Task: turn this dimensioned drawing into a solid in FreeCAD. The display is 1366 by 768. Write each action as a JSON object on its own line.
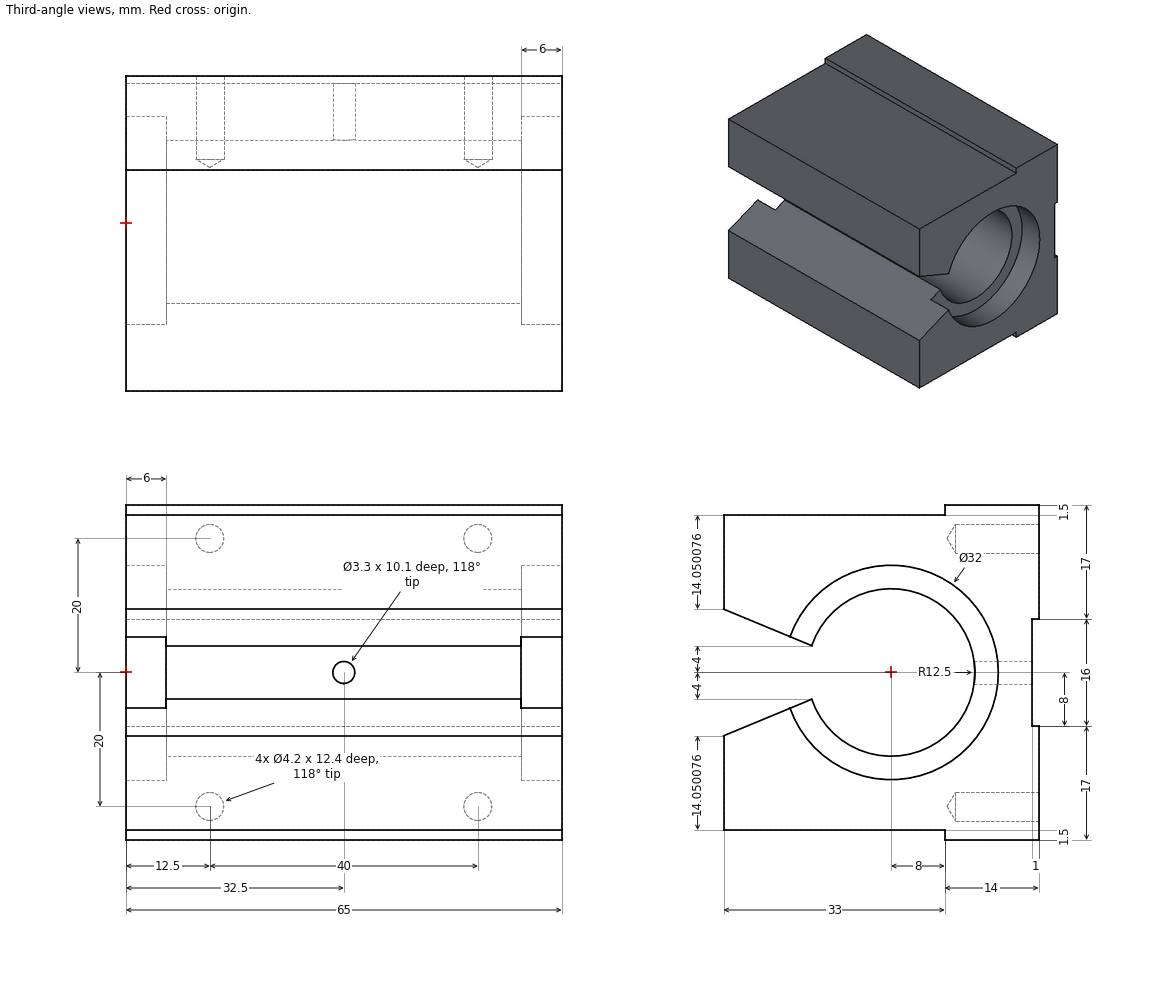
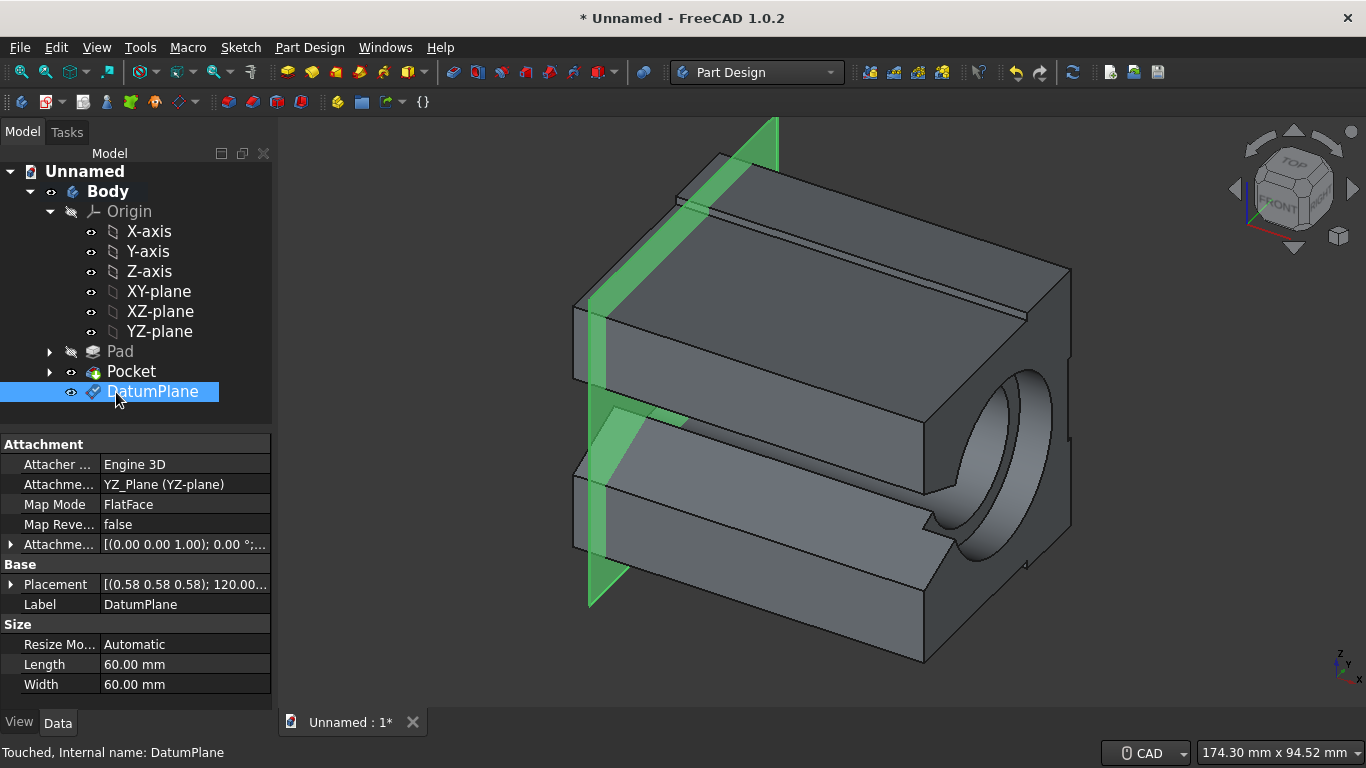
{"action": "left_click", "coordinate": [46, 102]}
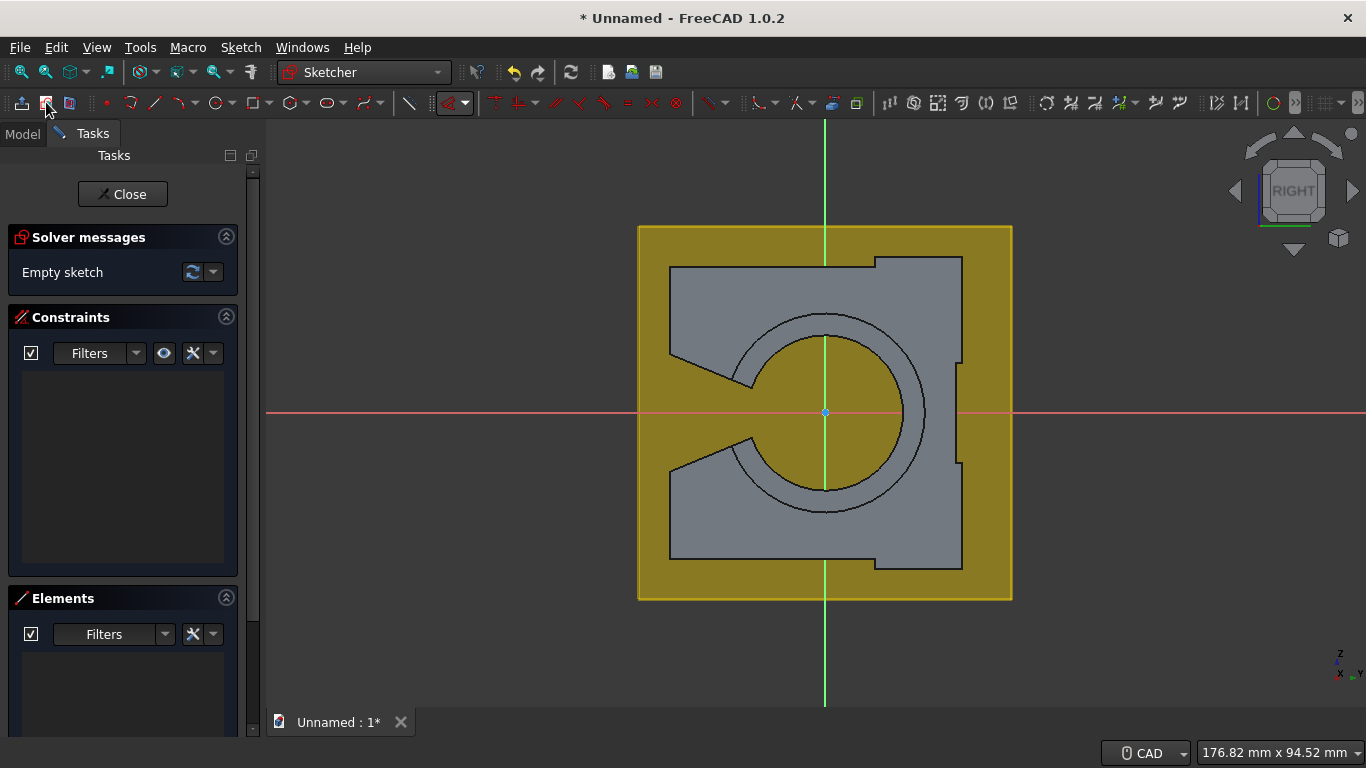
{"action": "key", "text": "q s"}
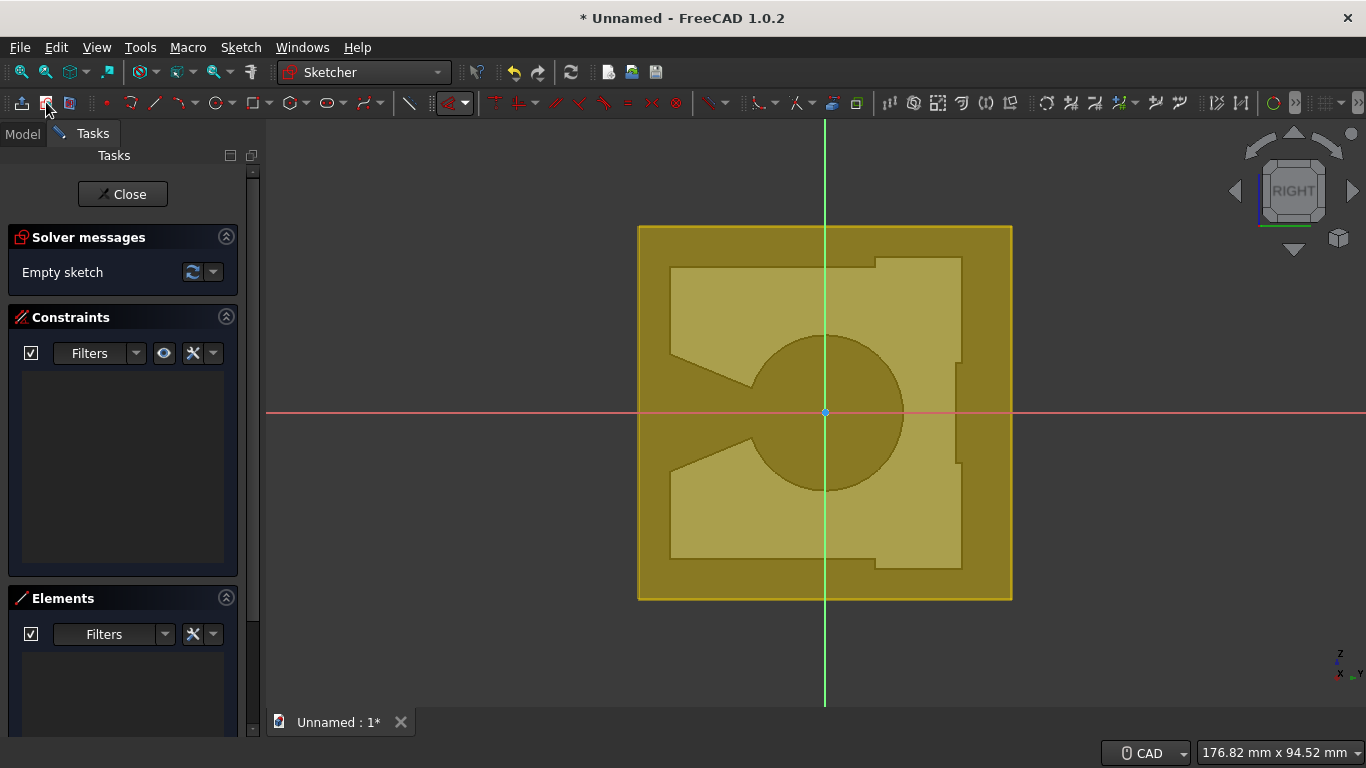
{"action": "scroll", "coordinate": [920, 413], "scroll_direction": "up", "scroll_amount": 3}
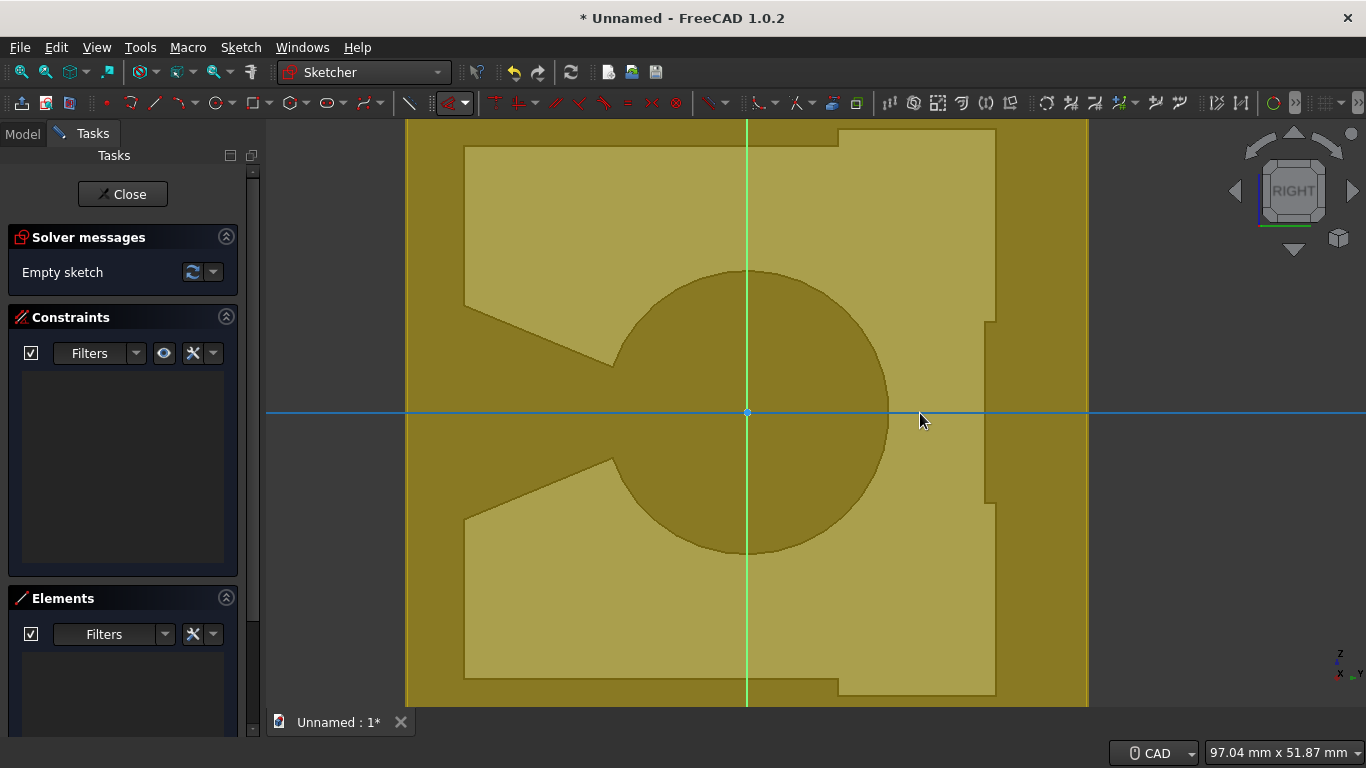
{"action": "key", "text": "g c"}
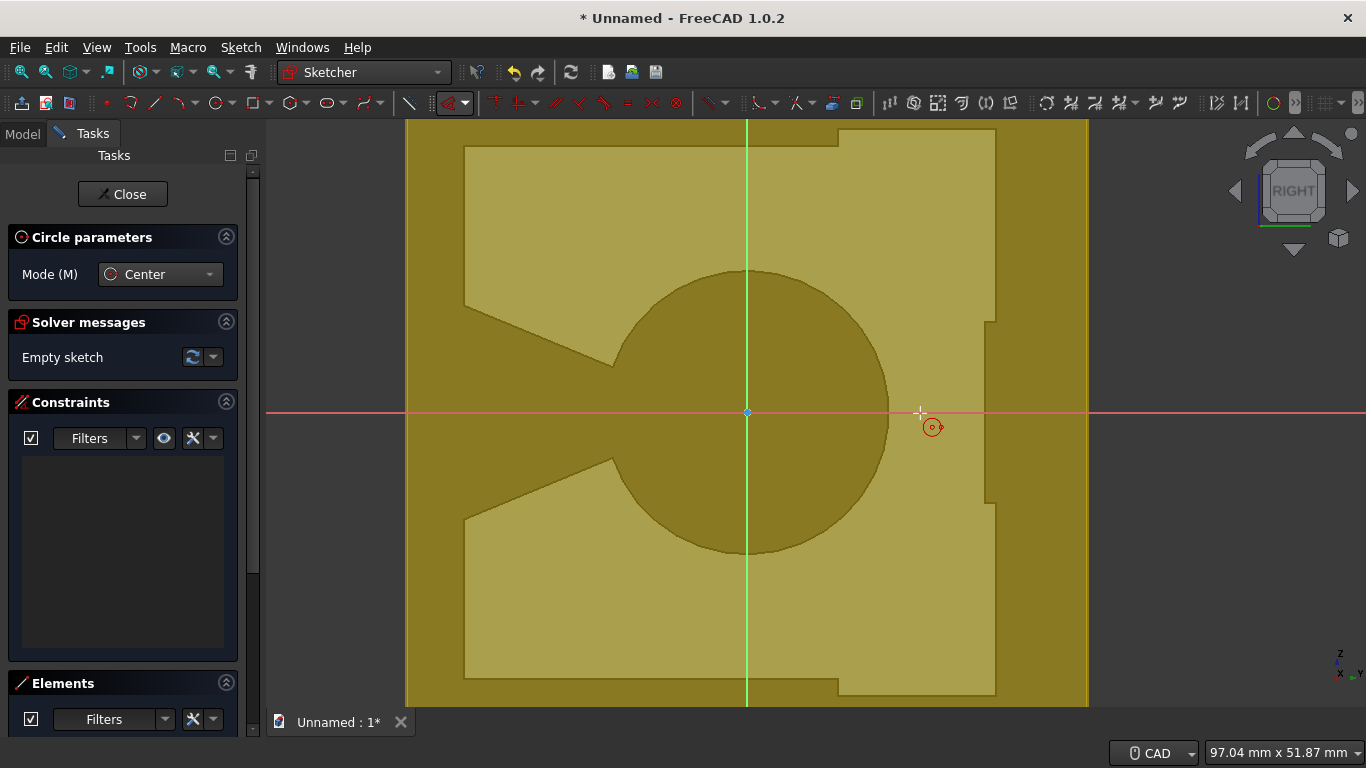
{"action": "left_click", "coordinate": [747, 413]}
{"action": "left_click", "coordinate": [875, 284]}
{"action": "key", "text": "Escape"}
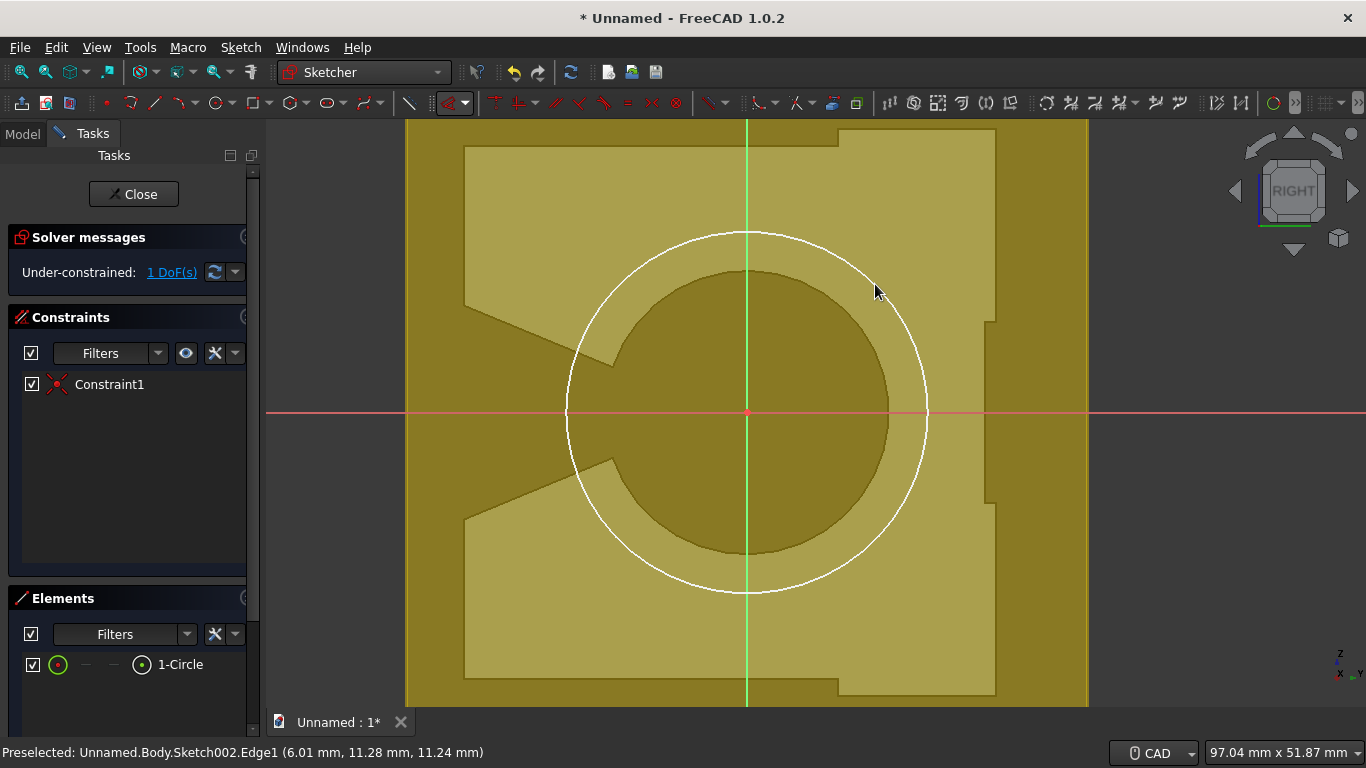
{"action": "left_click", "coordinate": [874, 284]}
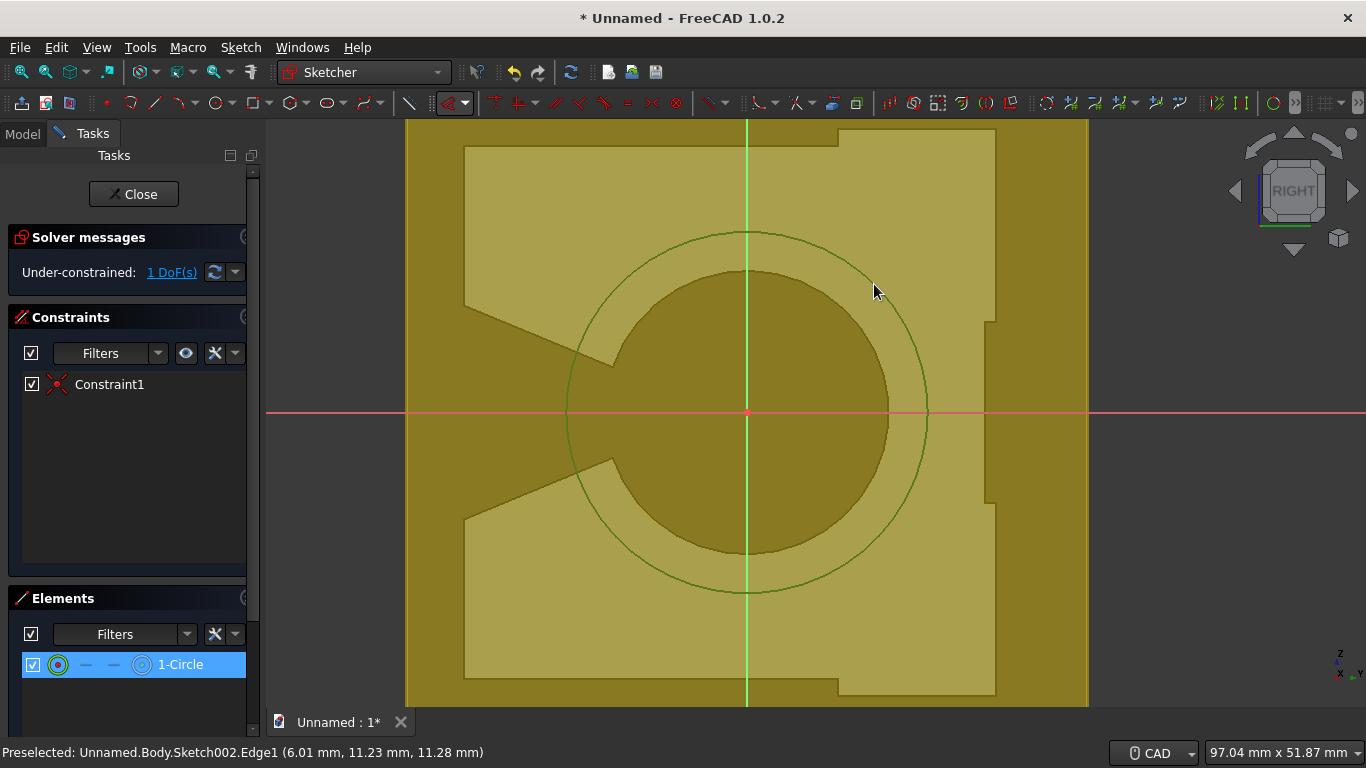
{"action": "key", "text": "k o"}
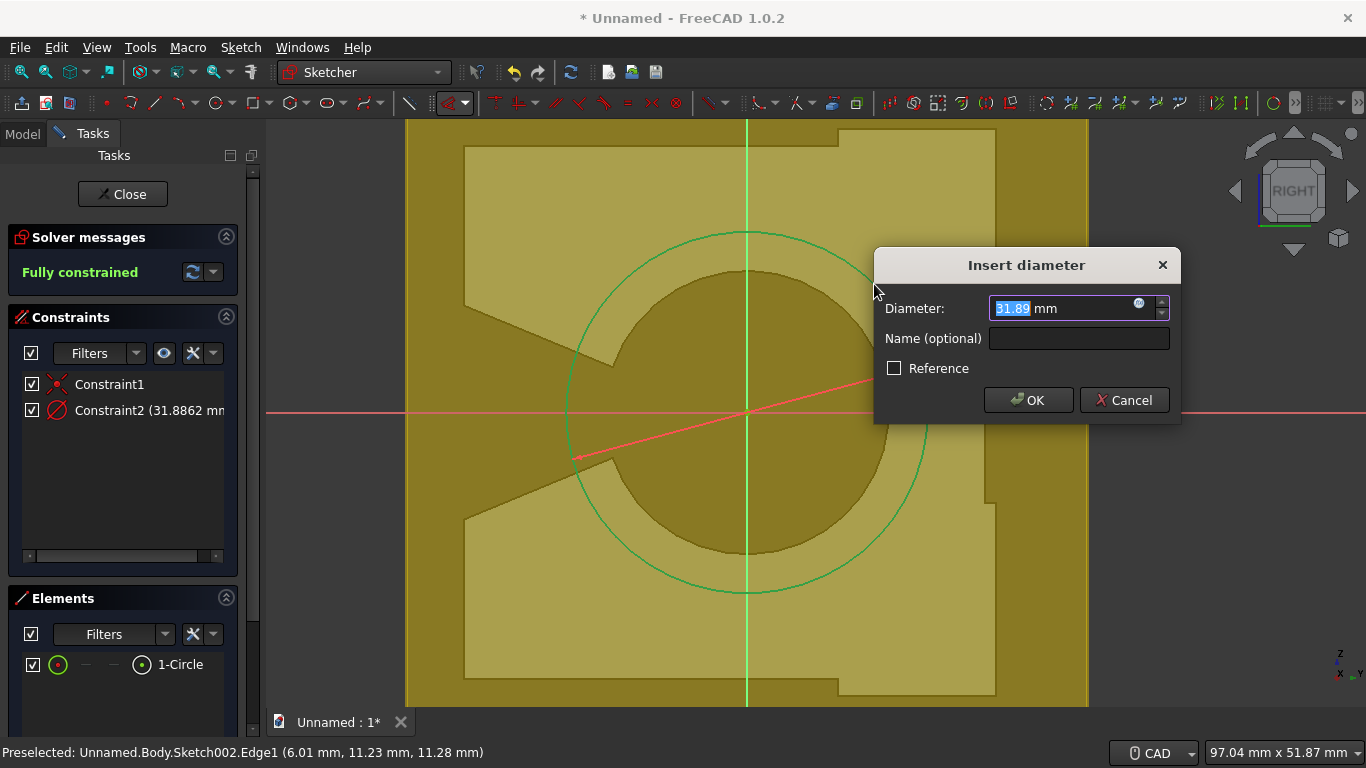
{"action": "type", "text": "32"}
{"action": "key", "text": "Return"}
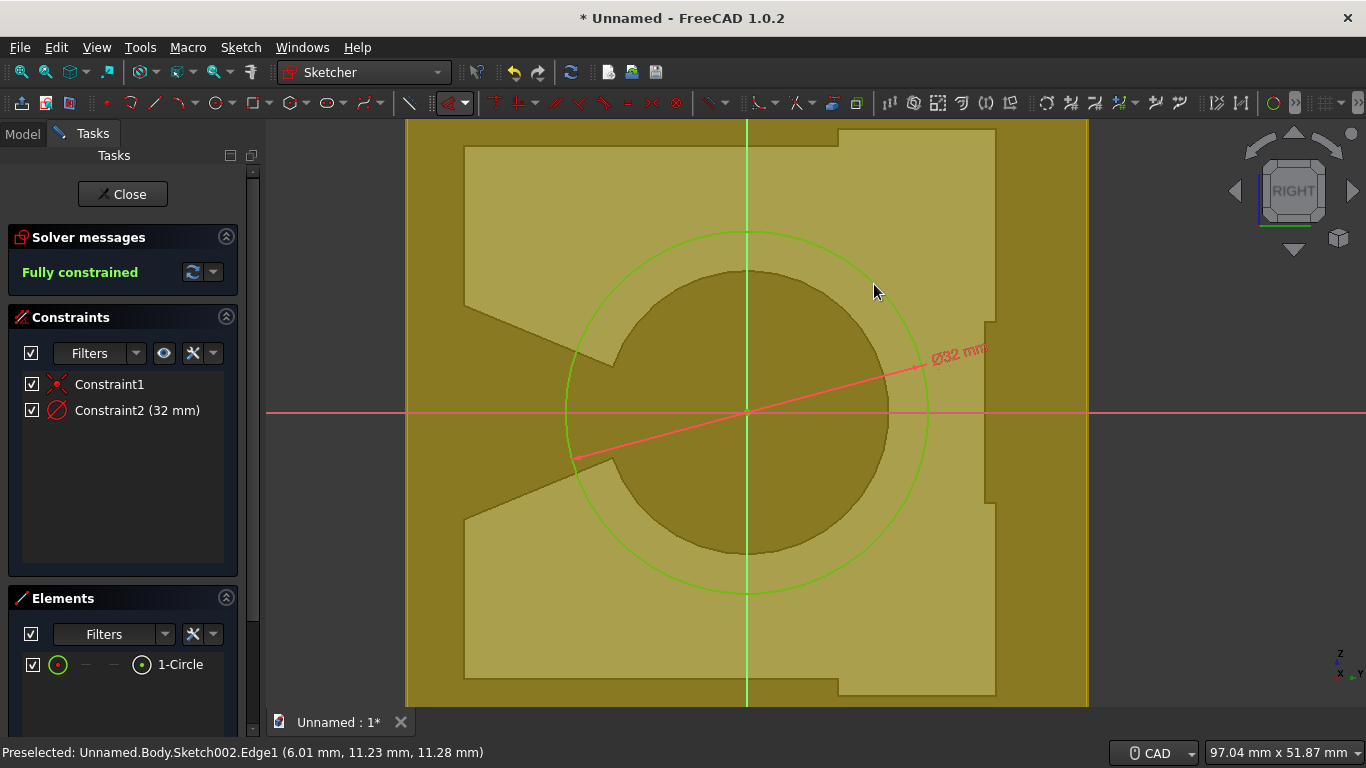
{"action": "left_click", "coordinate": [123, 194]}